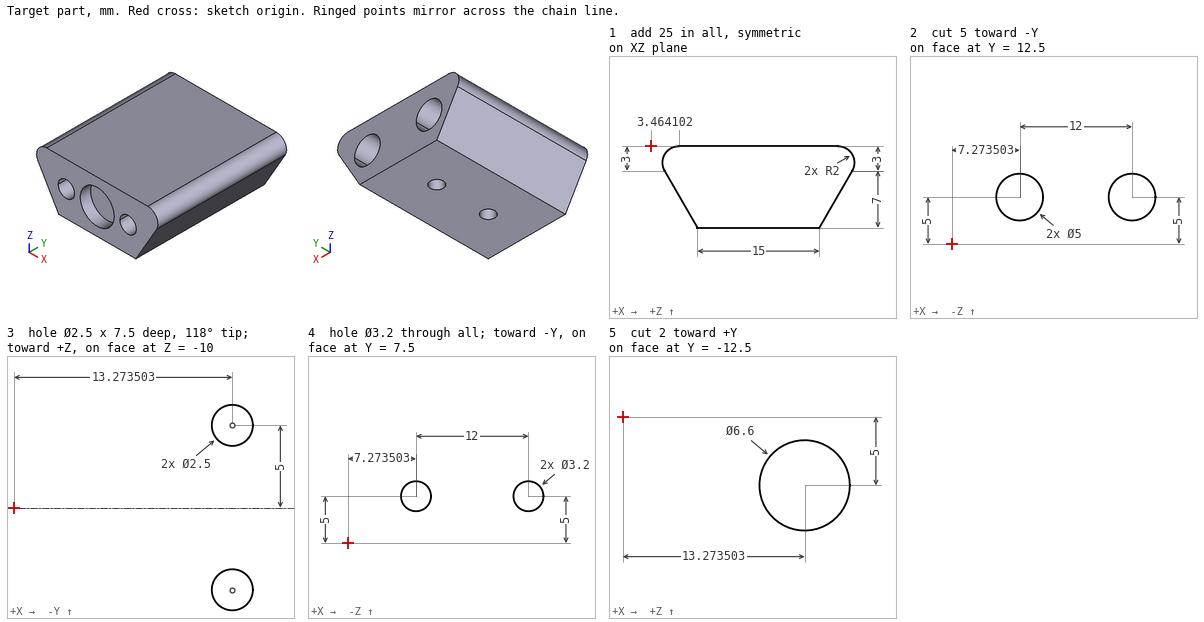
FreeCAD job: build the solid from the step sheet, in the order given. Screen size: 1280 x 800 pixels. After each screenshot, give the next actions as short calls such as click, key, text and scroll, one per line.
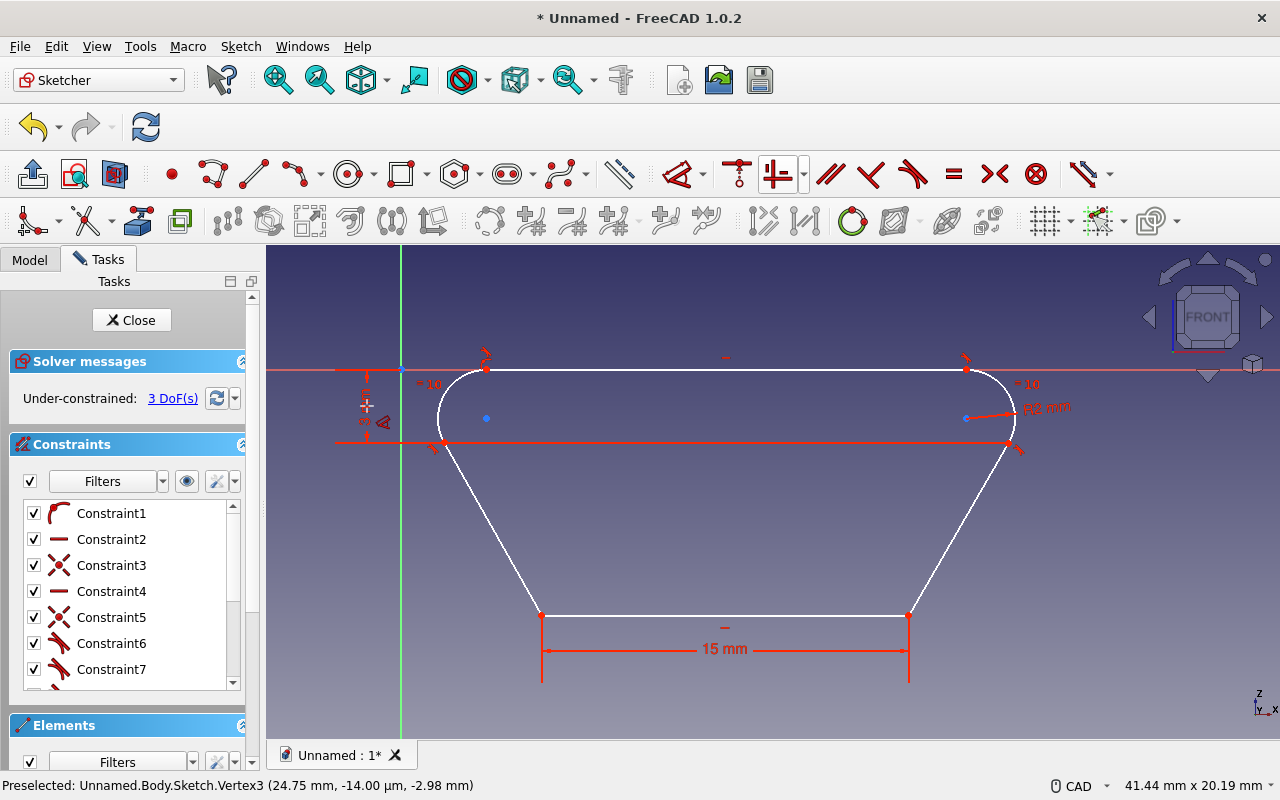
click(444, 443)
click(367, 432)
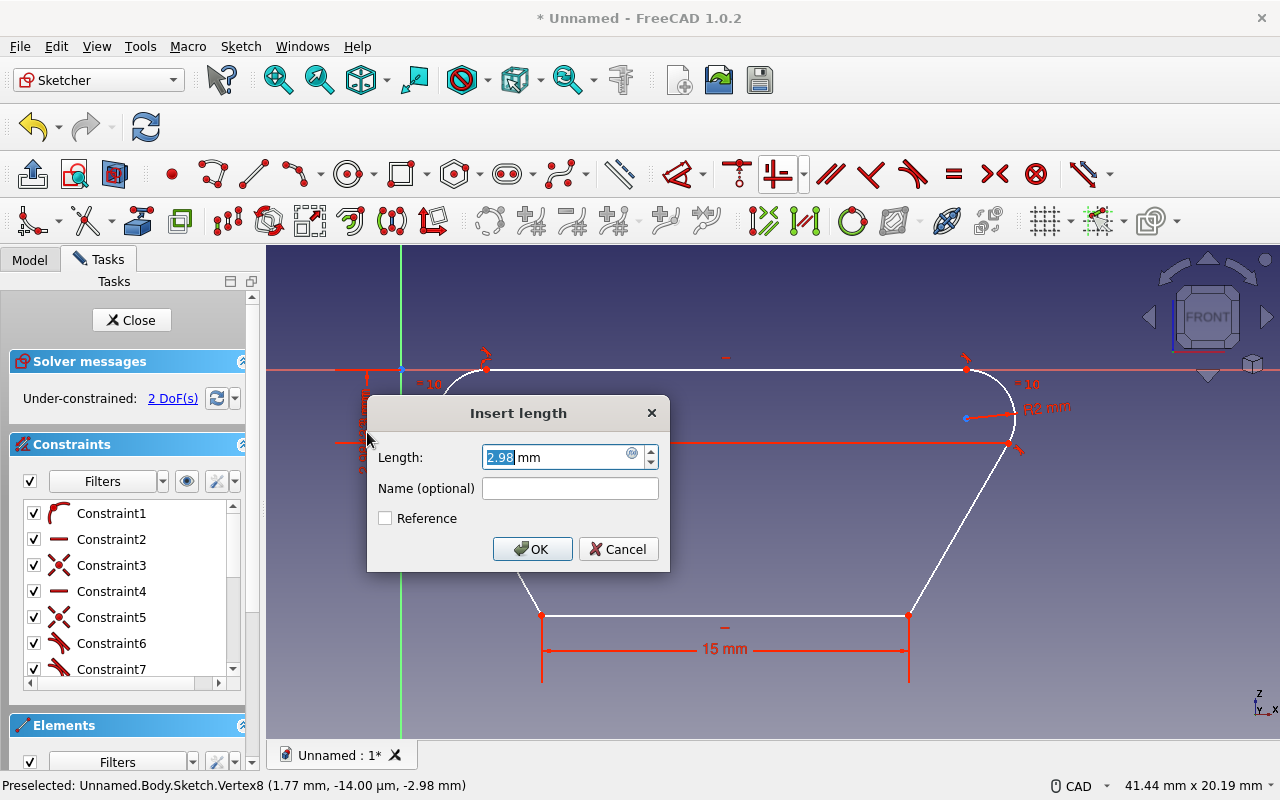
text(3)
key(Return)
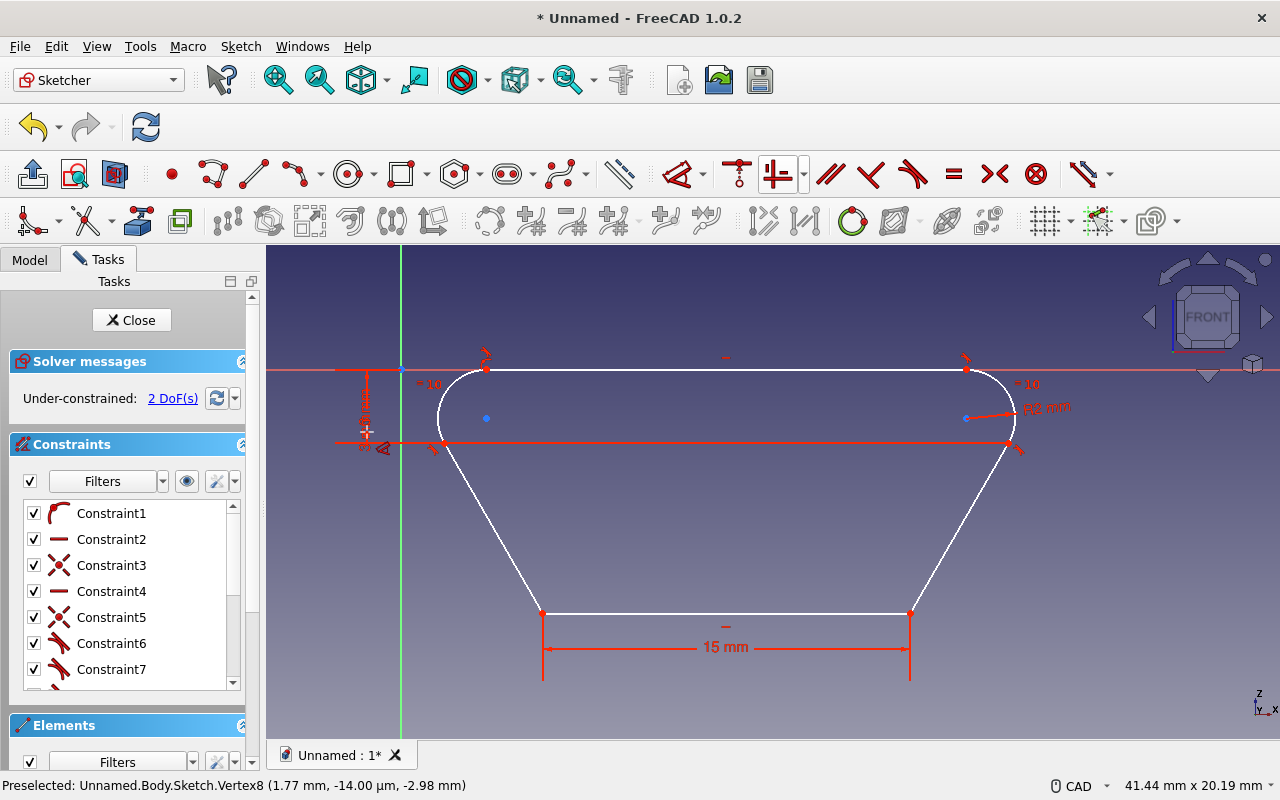
click(979, 494)
click(1042, 529)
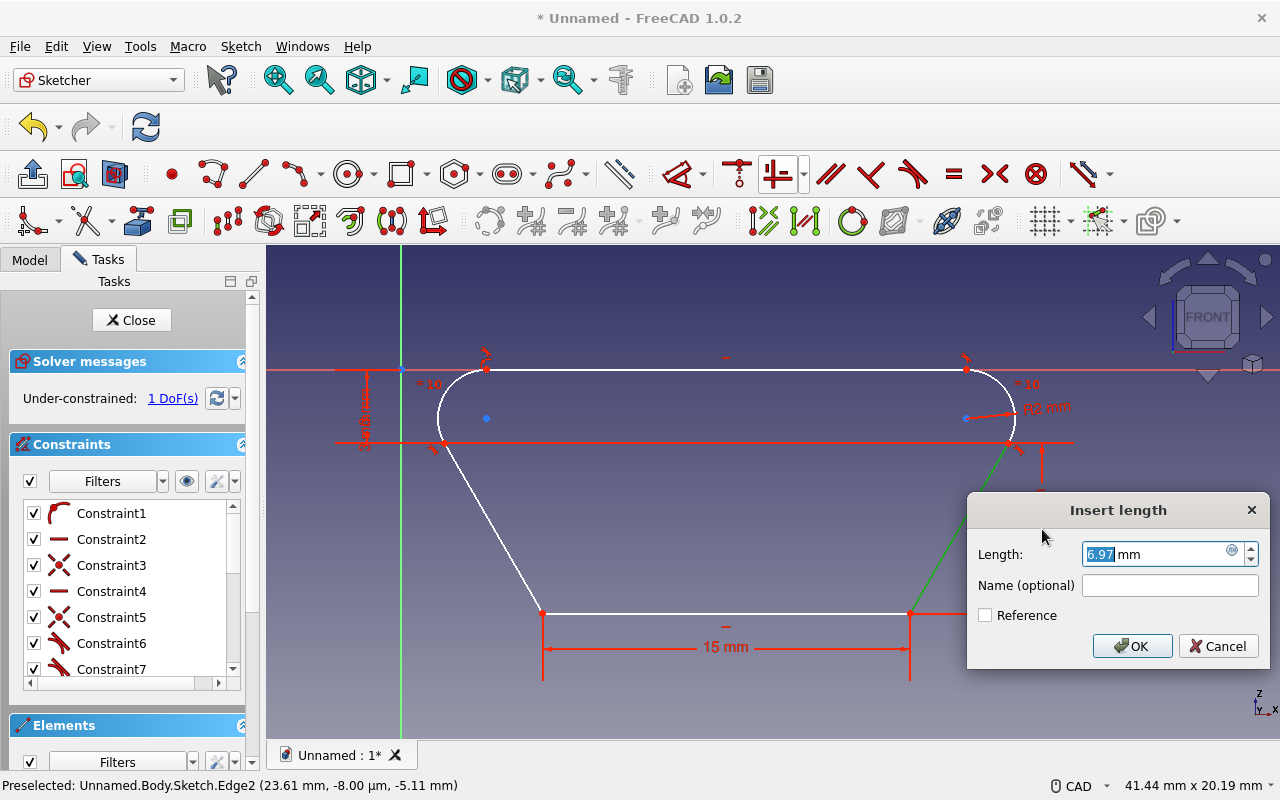
text(7)
key(Return)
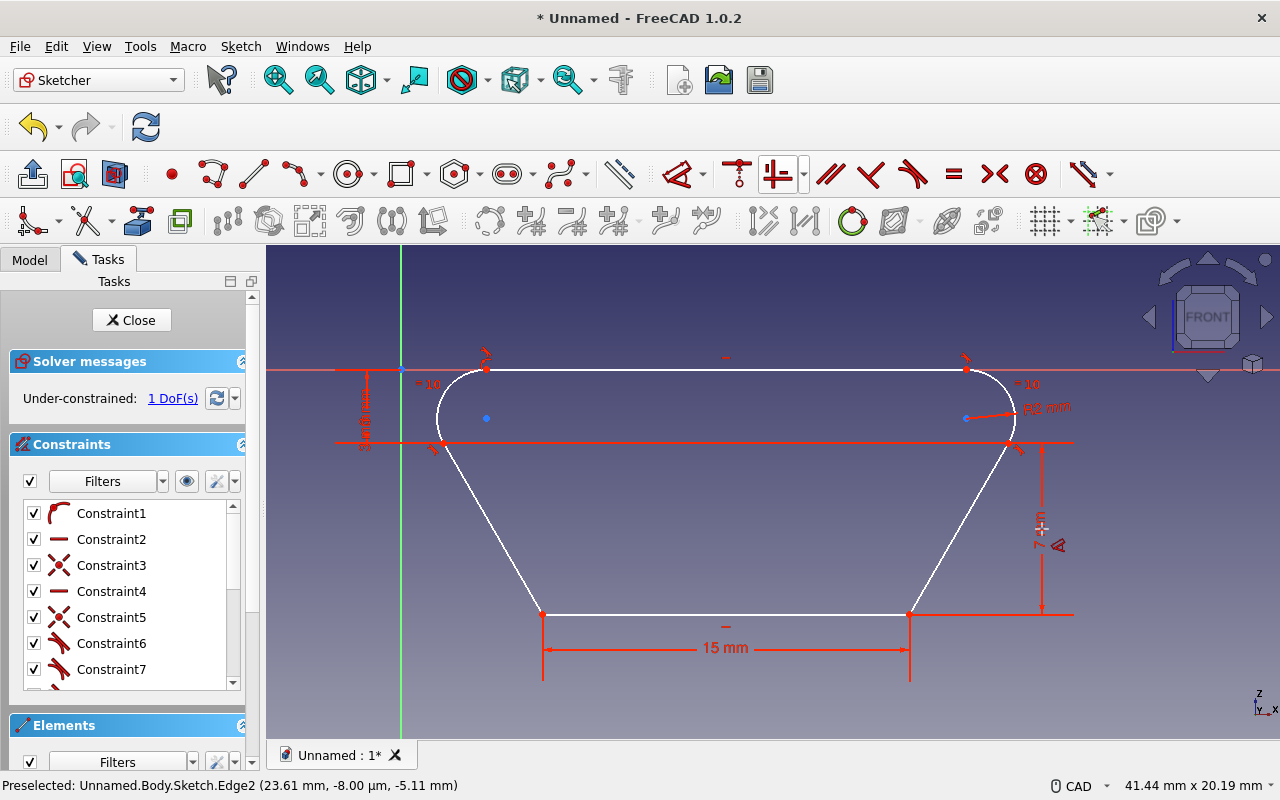
click(486, 370)
click(444, 336)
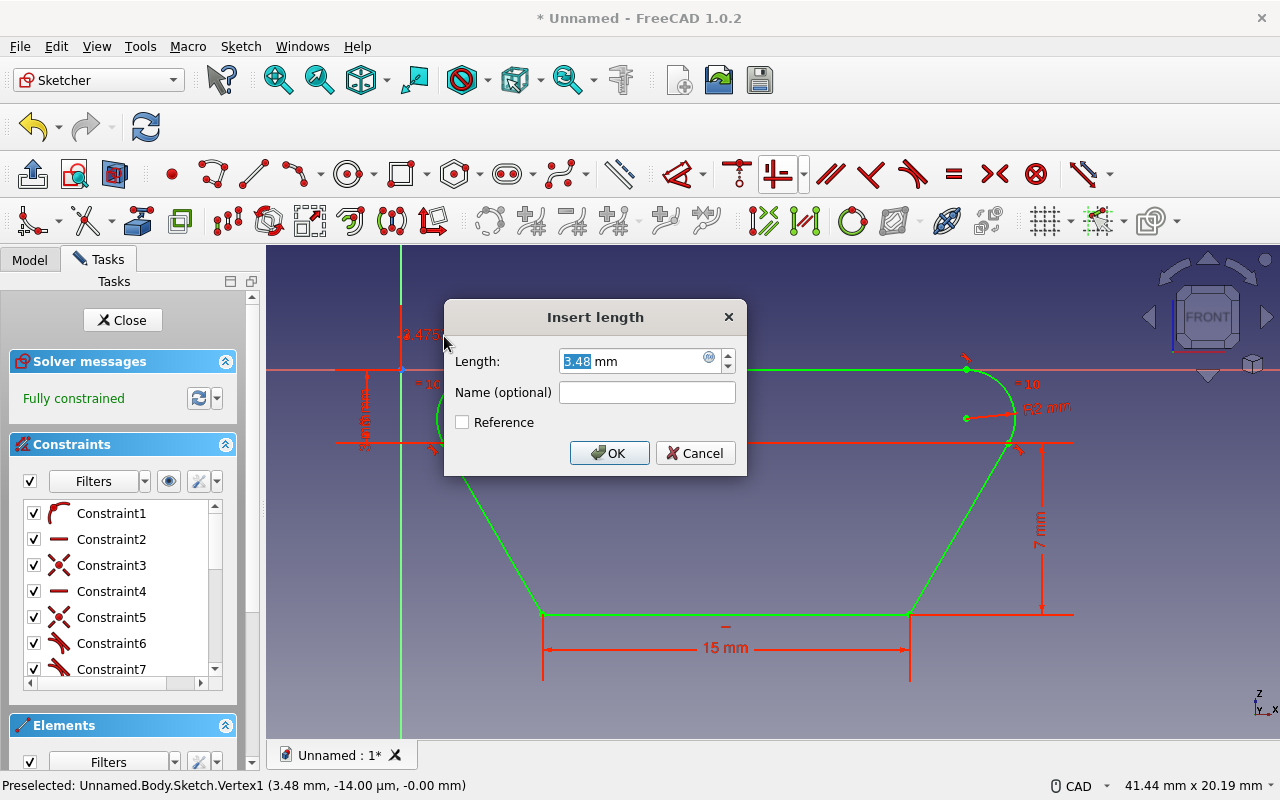
text(3.464102)
key(Return)
key(Escape)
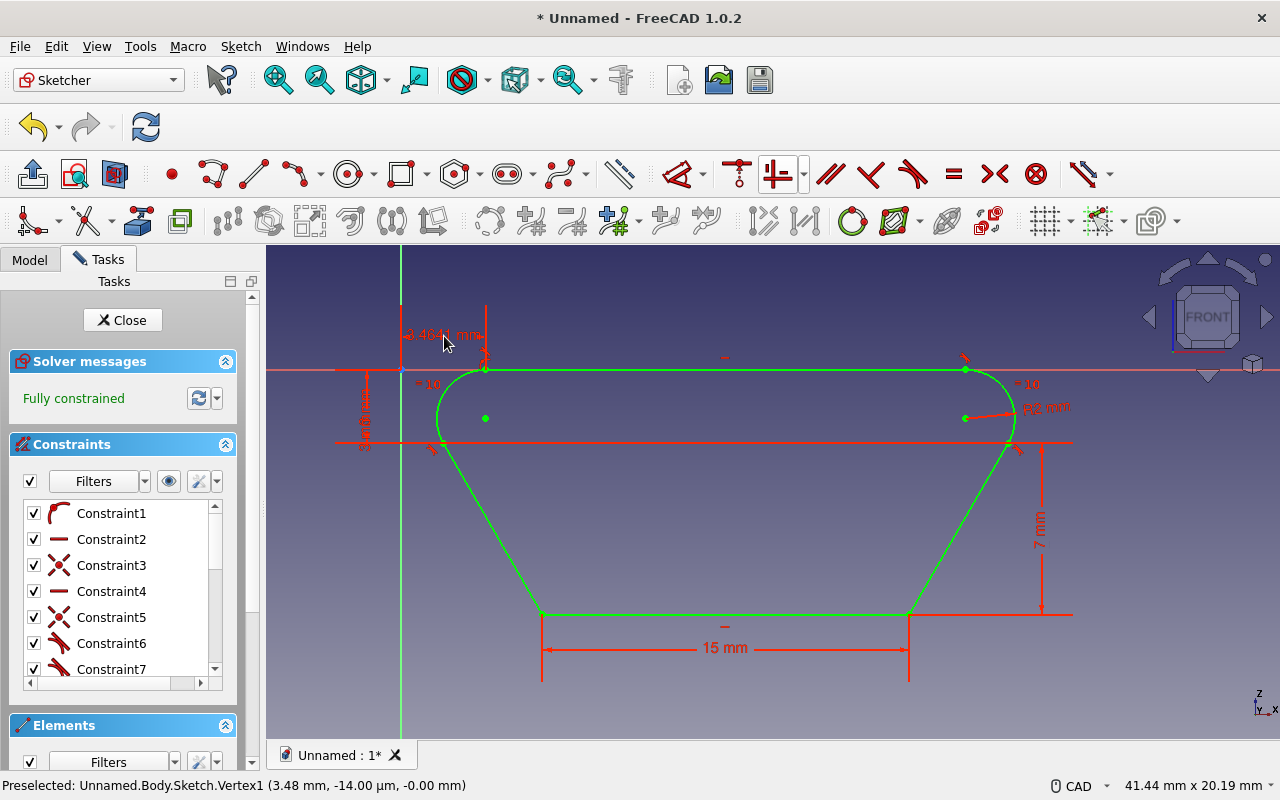
click(123, 320)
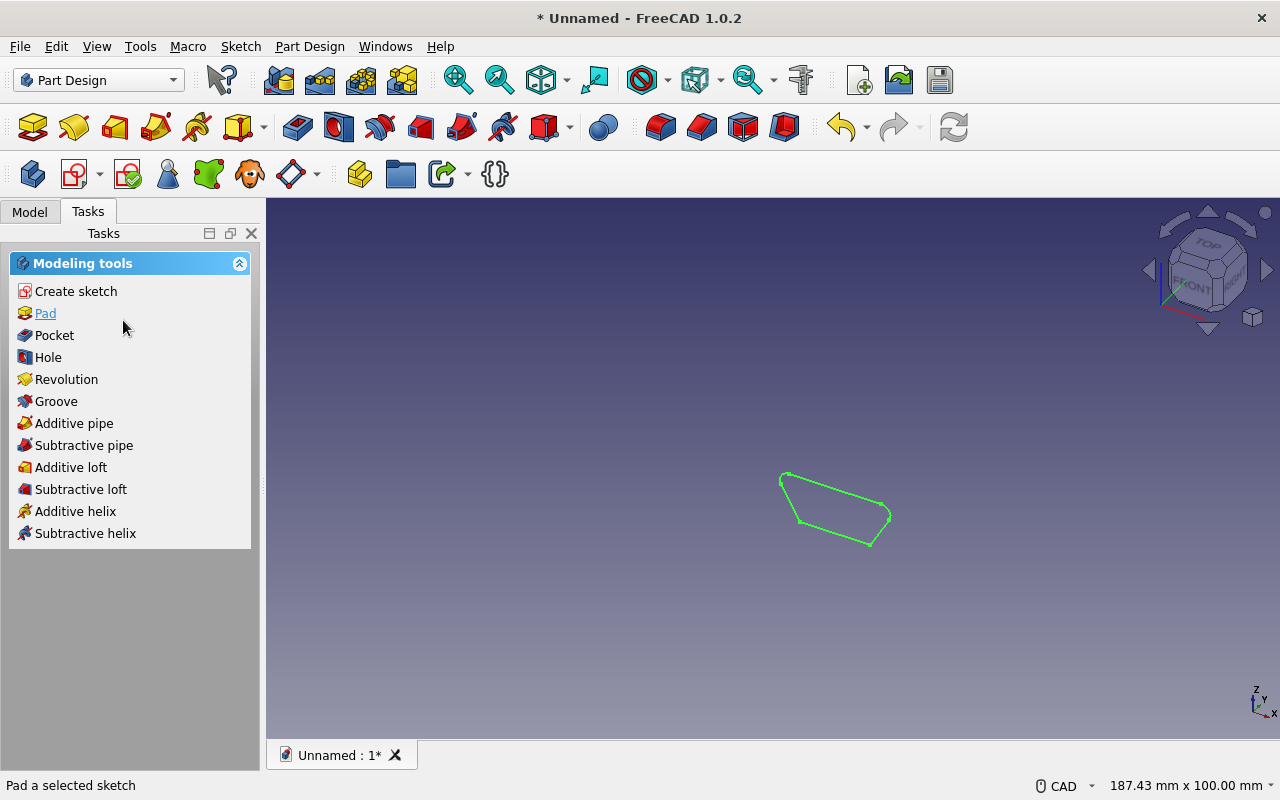
click(33, 128)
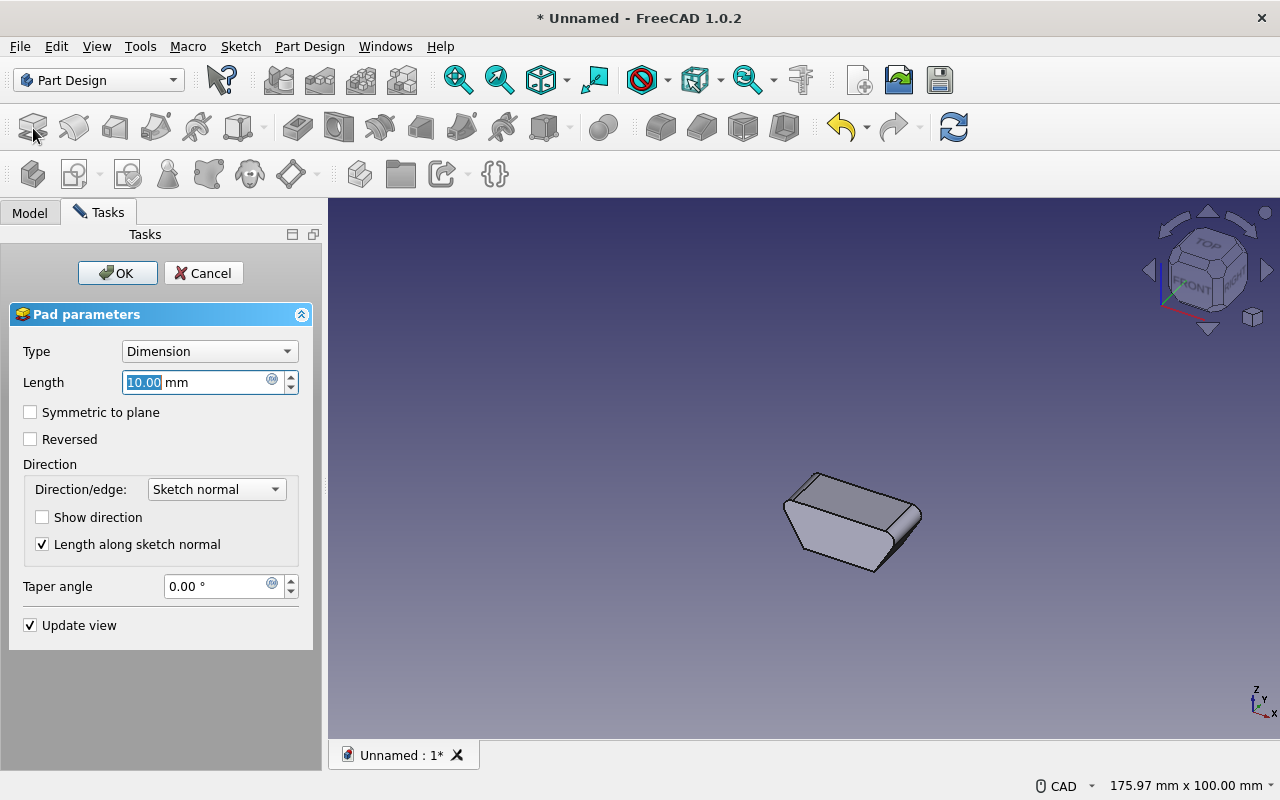
text(25)
key(Tab)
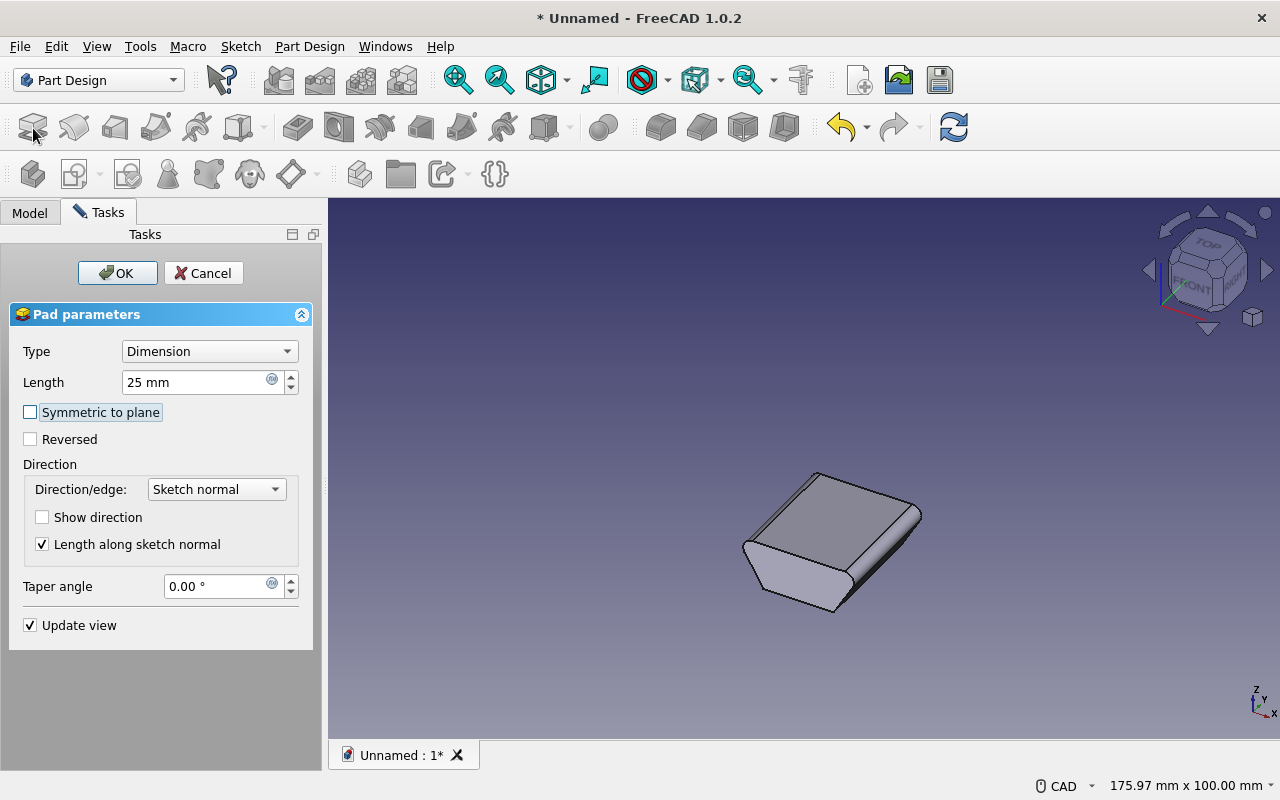
click(31, 412)